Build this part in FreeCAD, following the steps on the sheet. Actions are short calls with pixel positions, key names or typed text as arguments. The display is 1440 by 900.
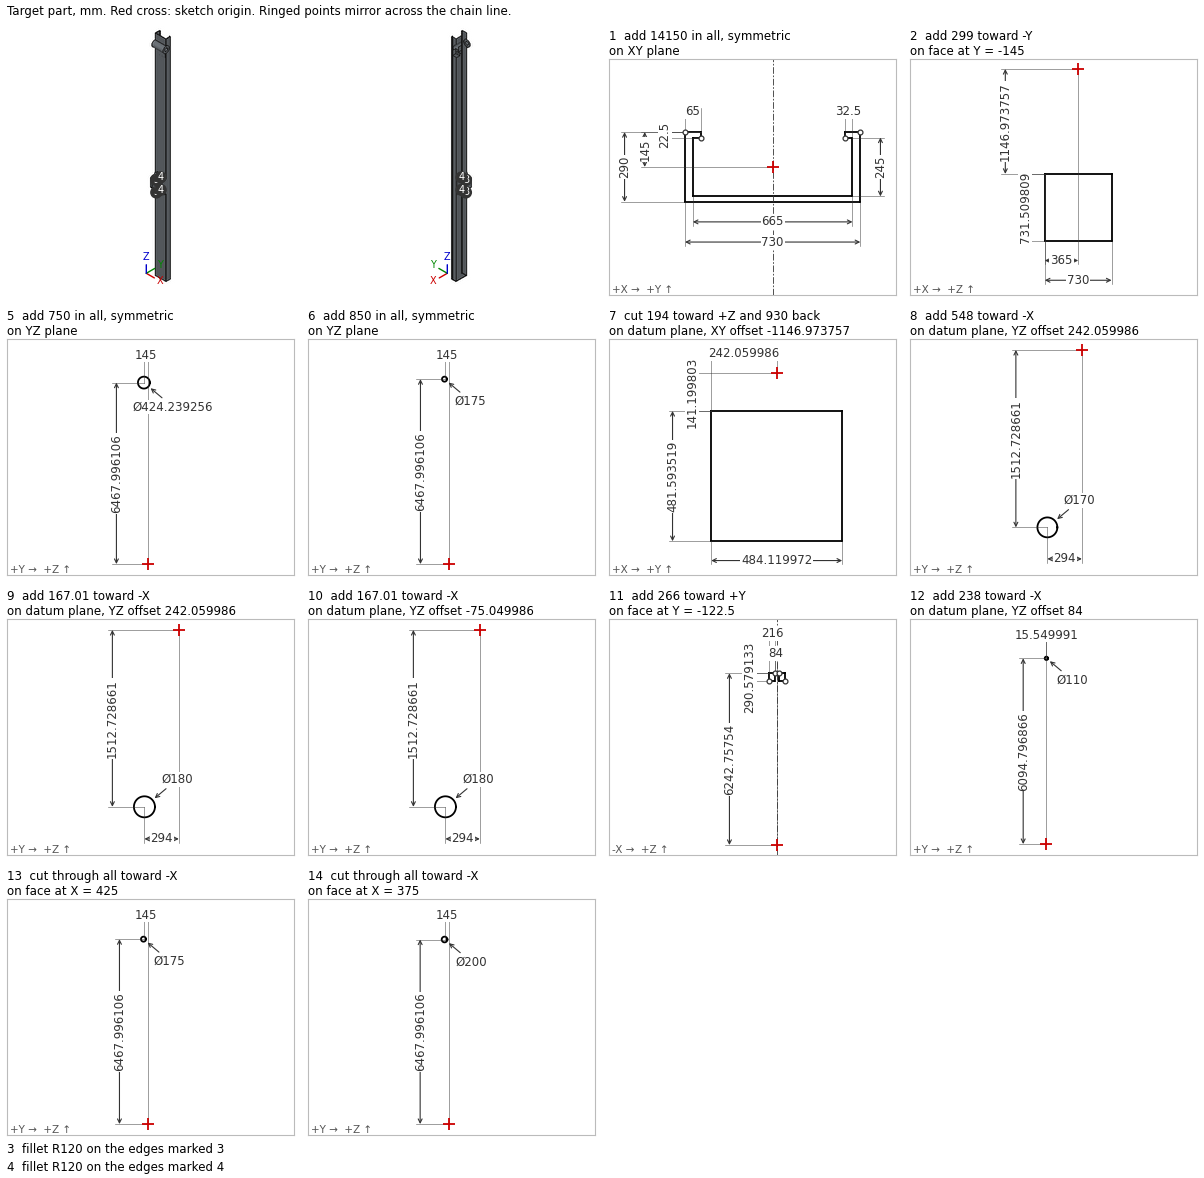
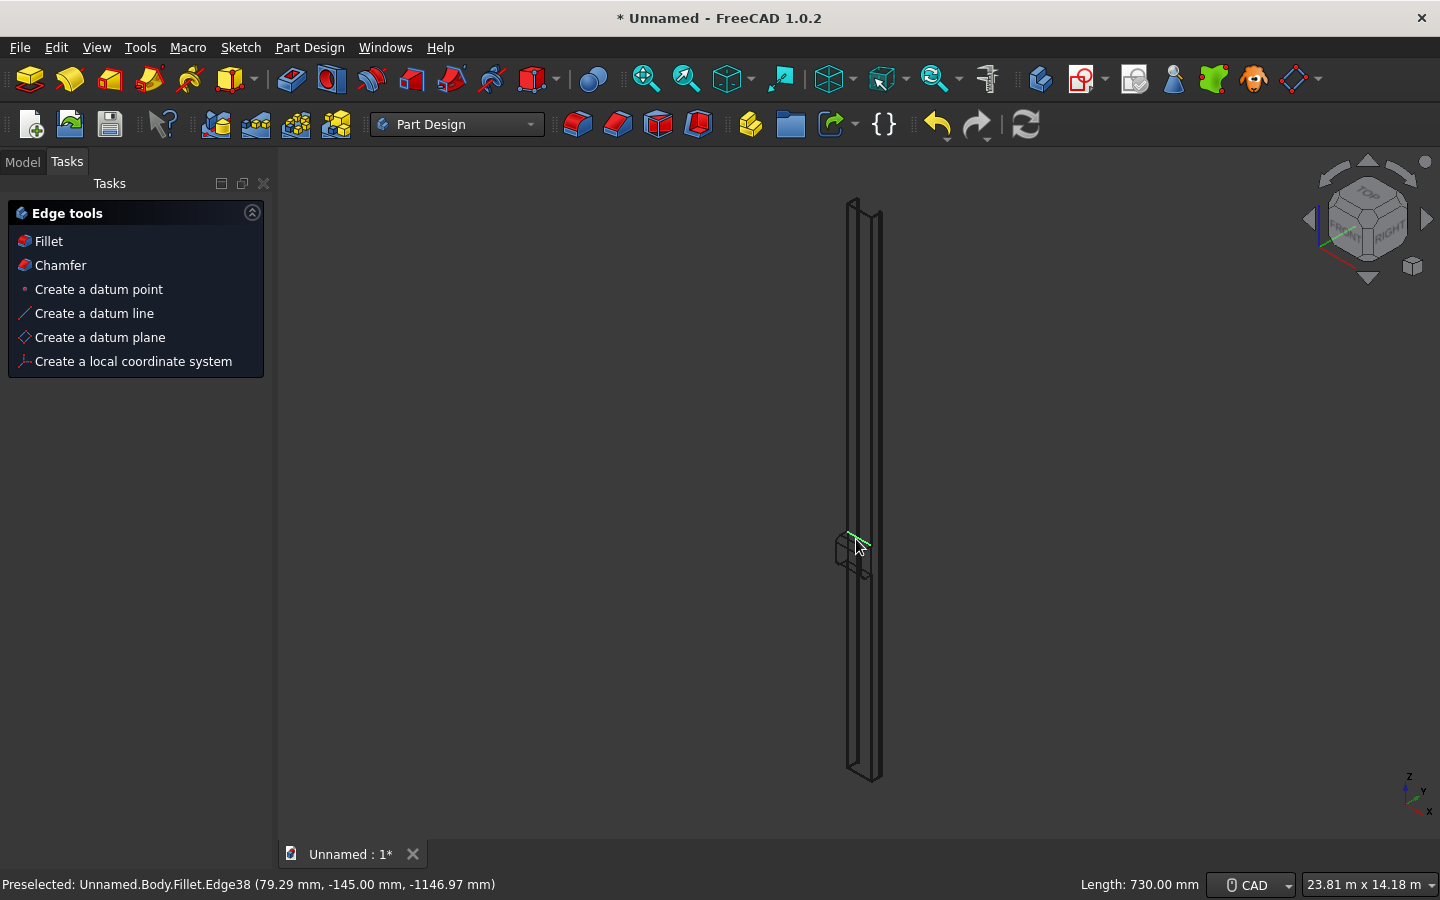
click(852, 562, ctrl)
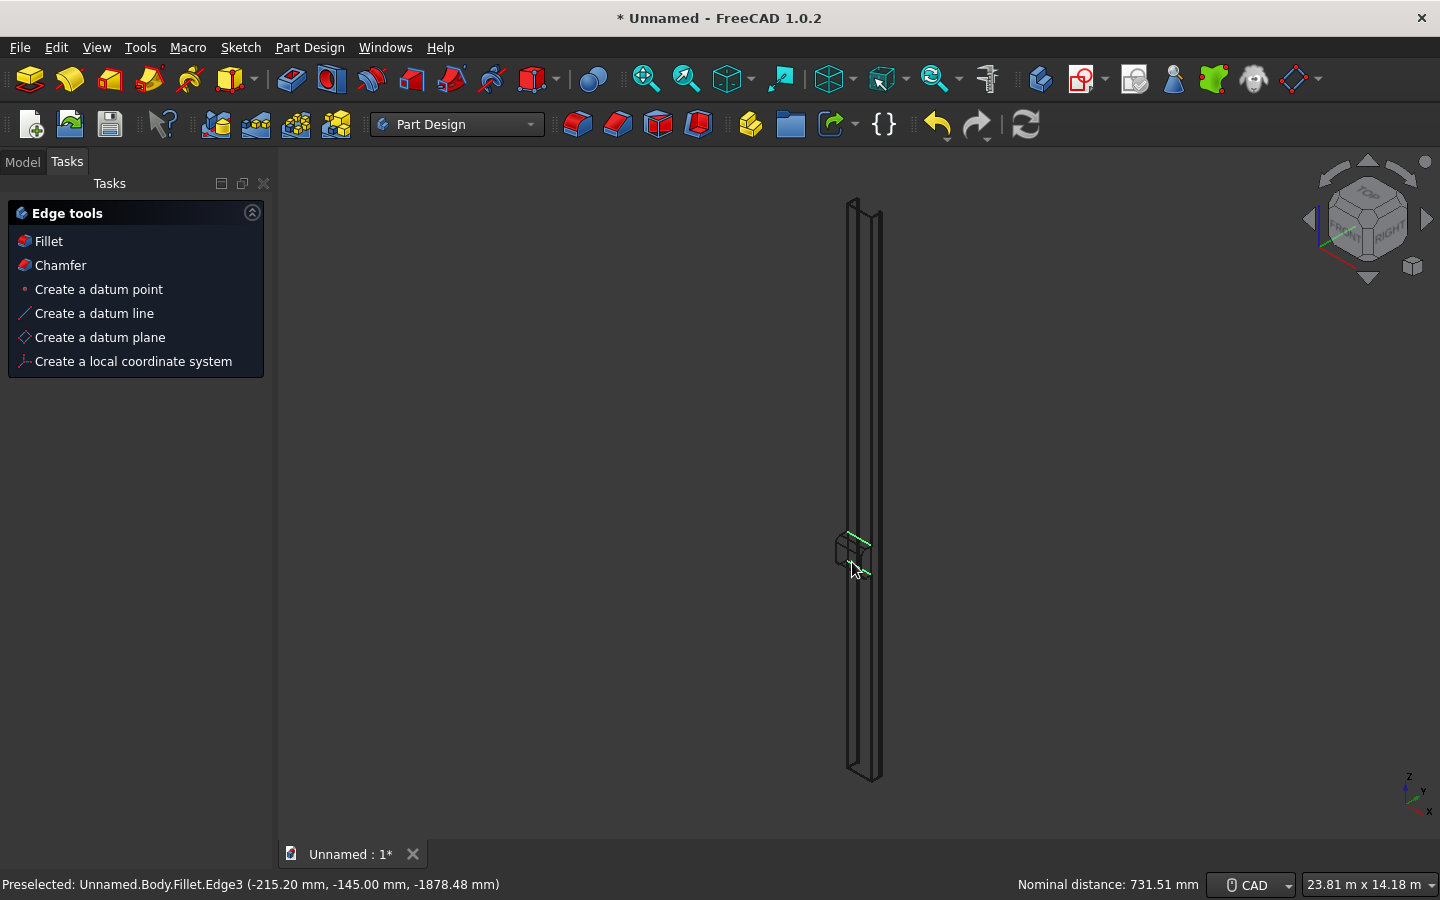
key(v)
key(1)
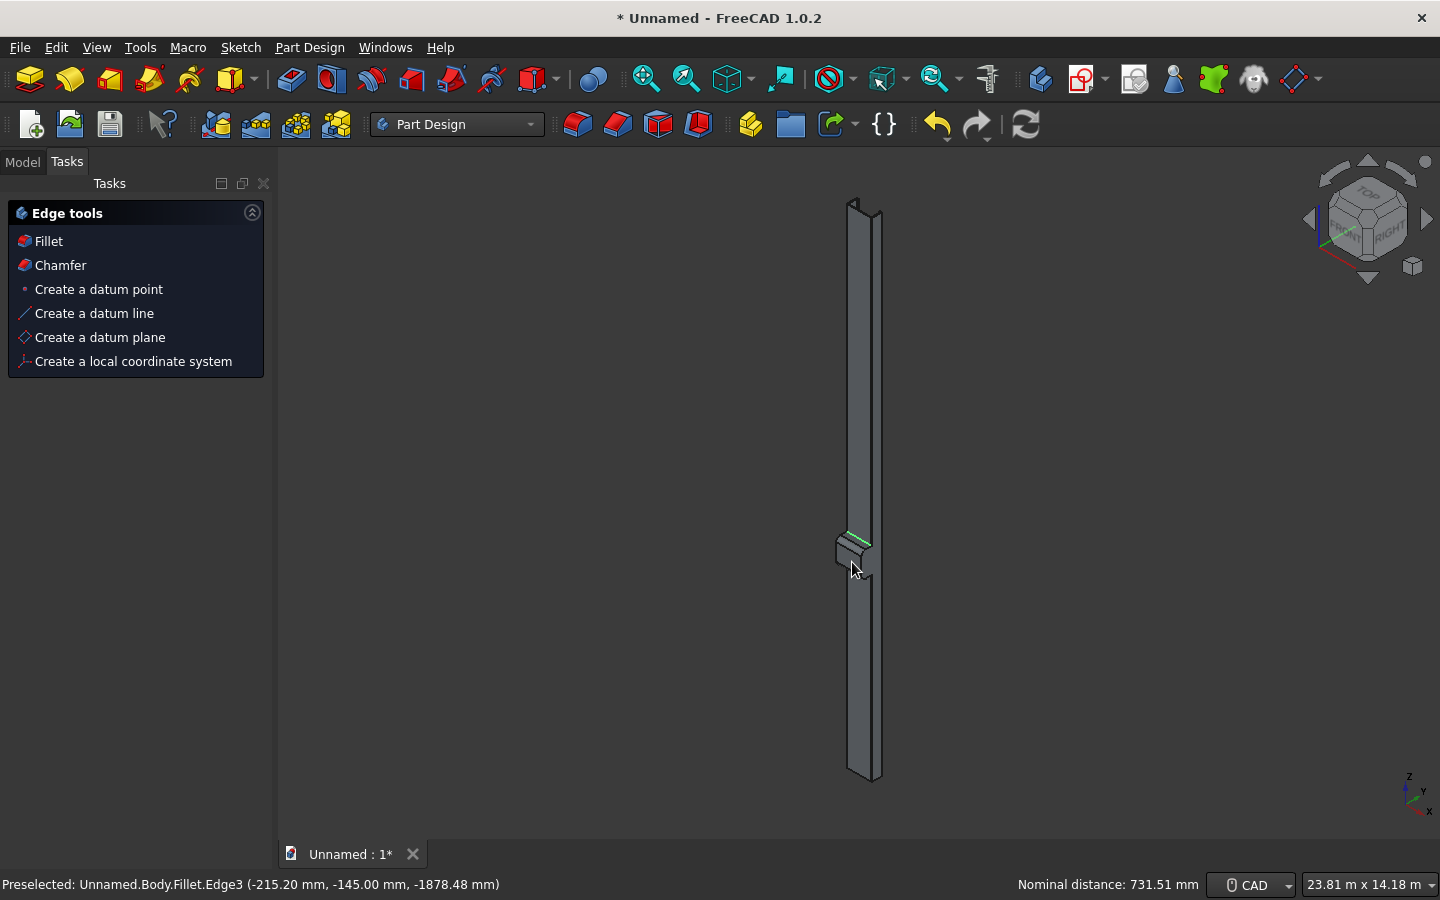
click(578, 124)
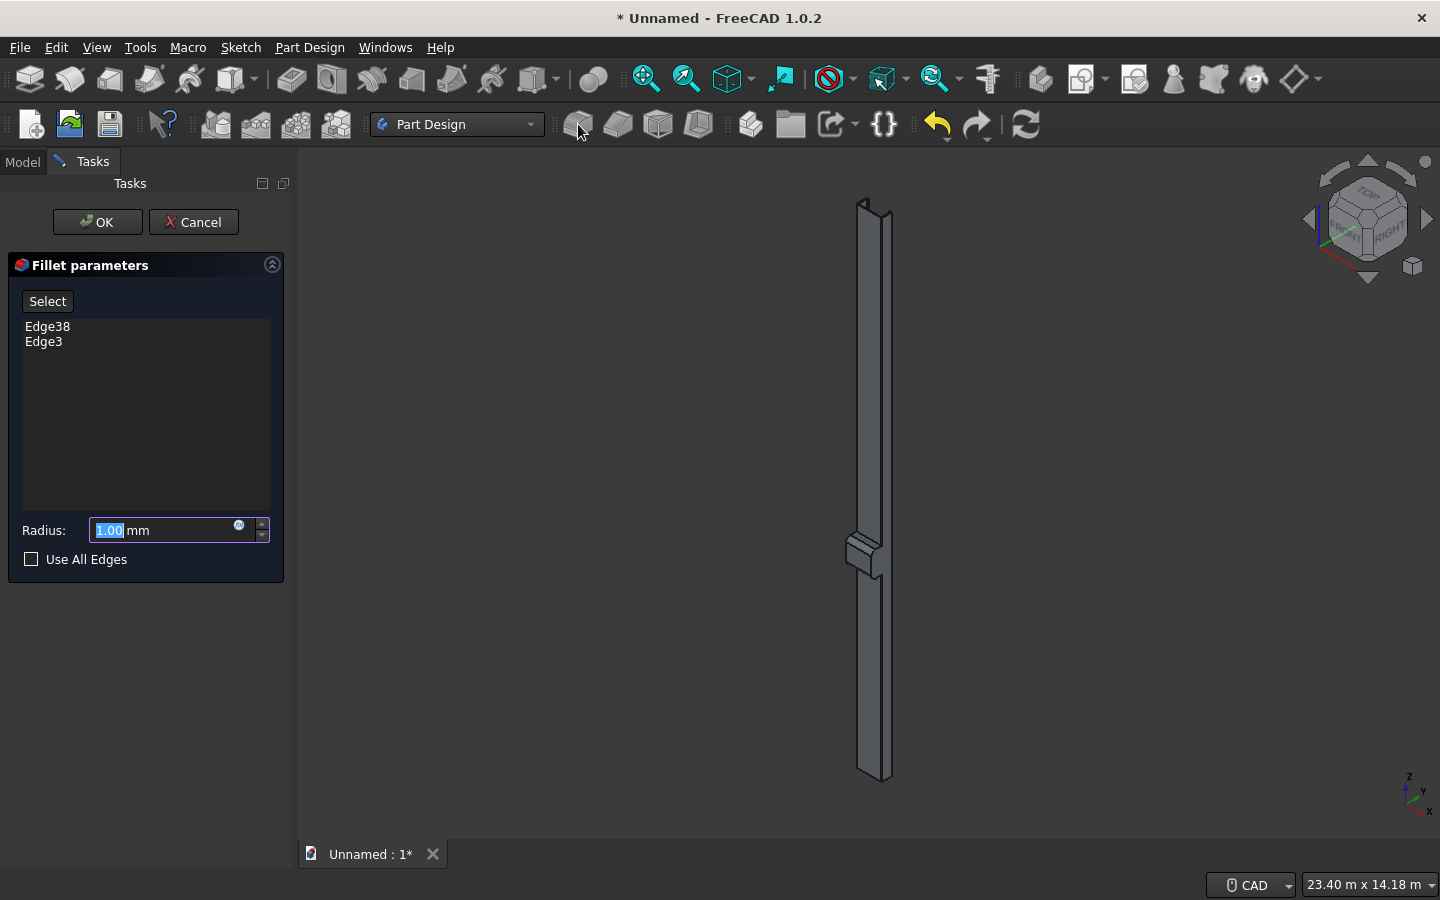
text(120)
key(Tab)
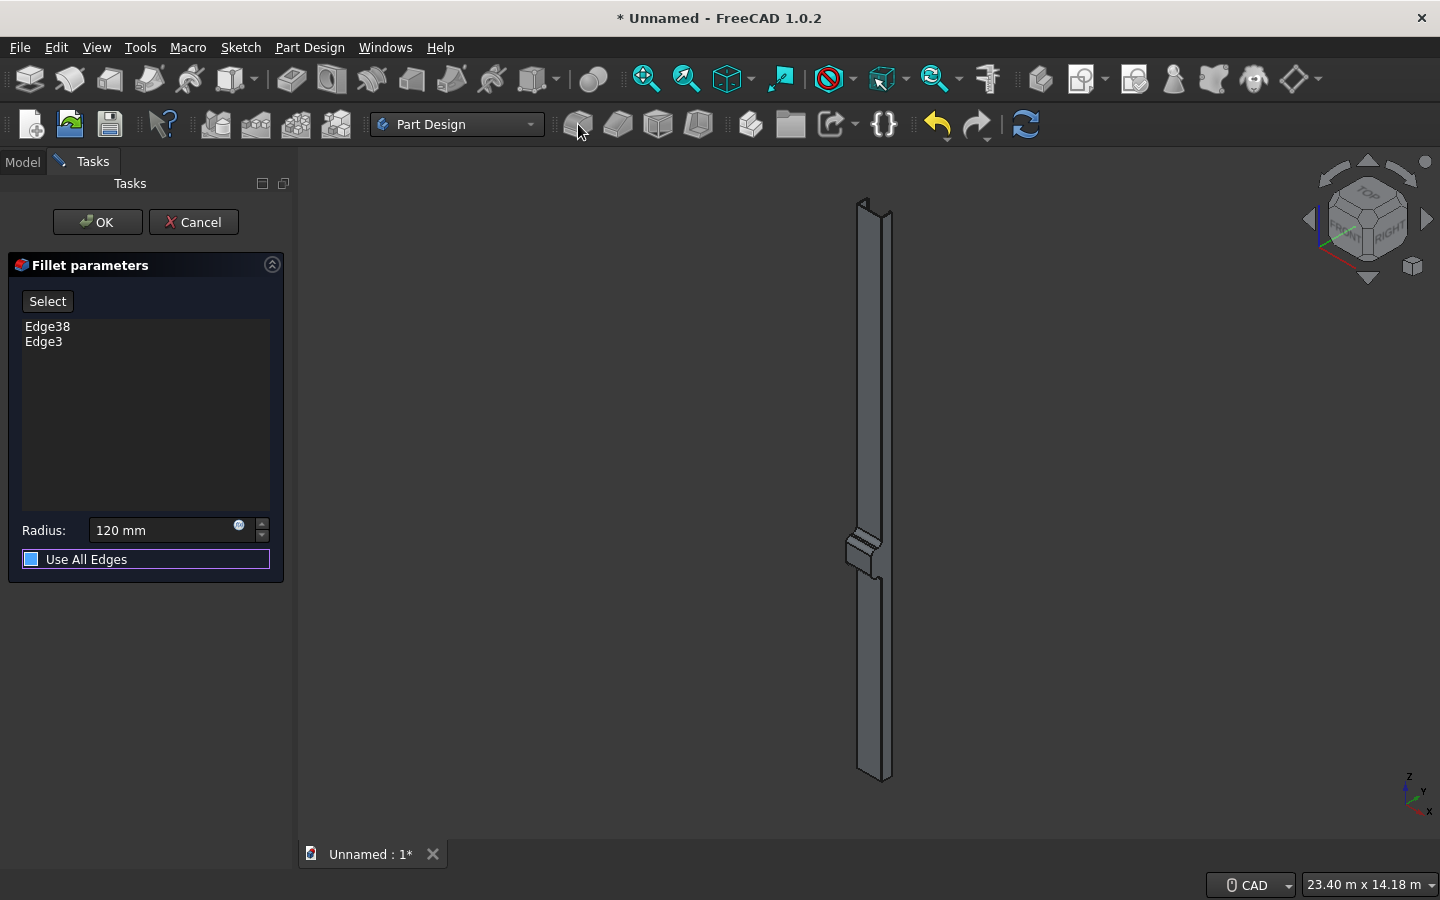
click(98, 222)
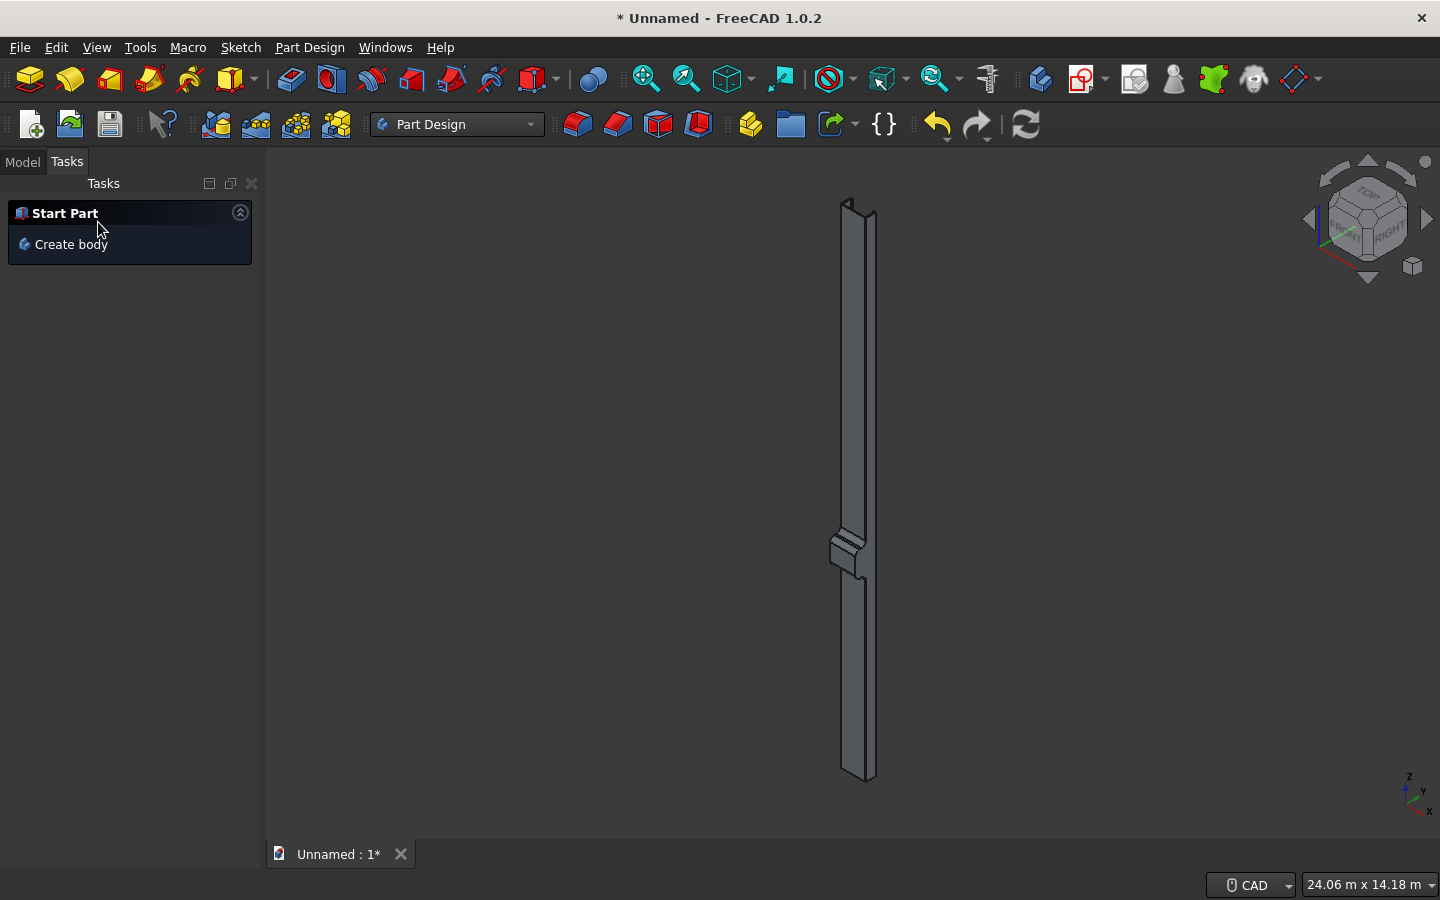
click(1082, 80)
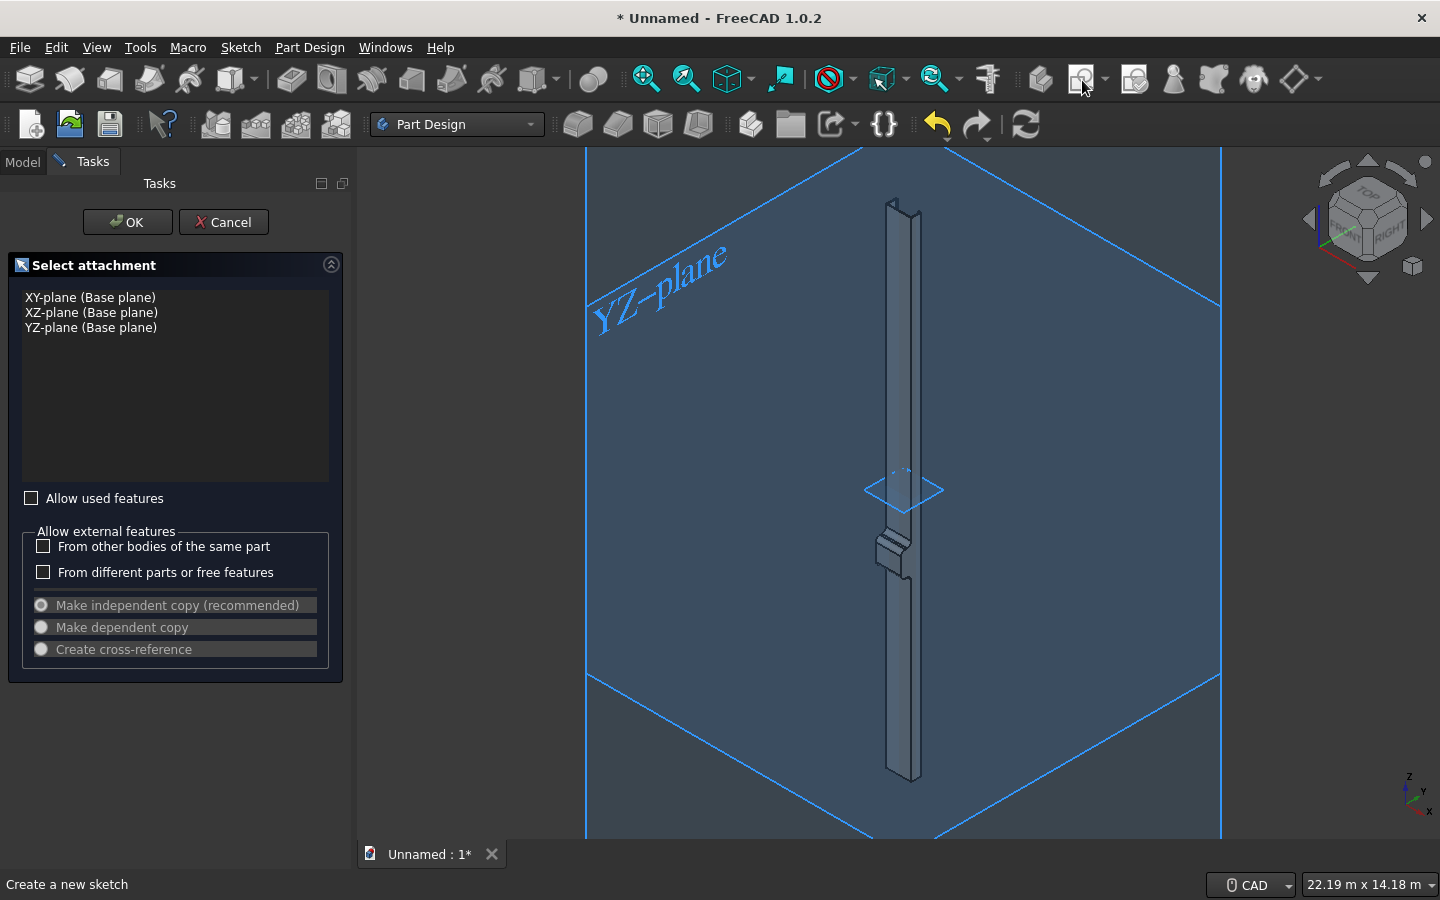
click(82, 328)